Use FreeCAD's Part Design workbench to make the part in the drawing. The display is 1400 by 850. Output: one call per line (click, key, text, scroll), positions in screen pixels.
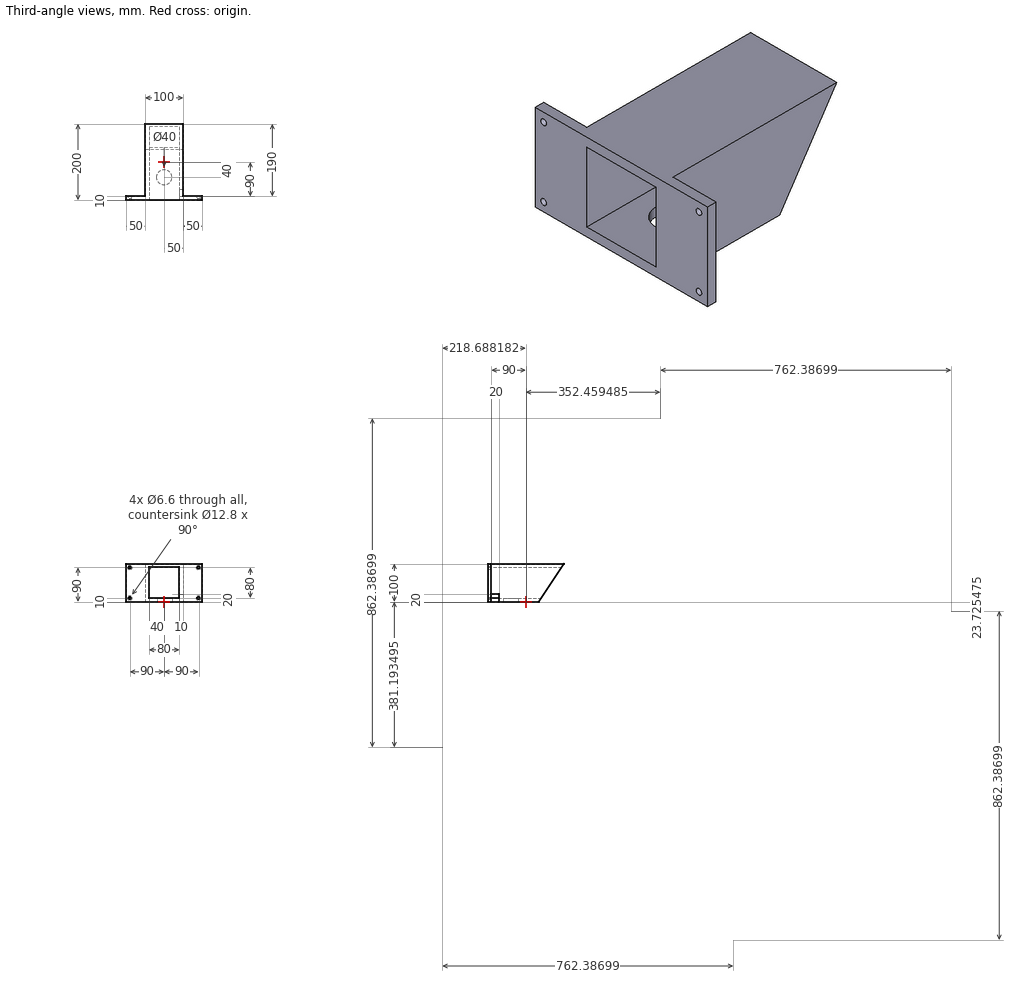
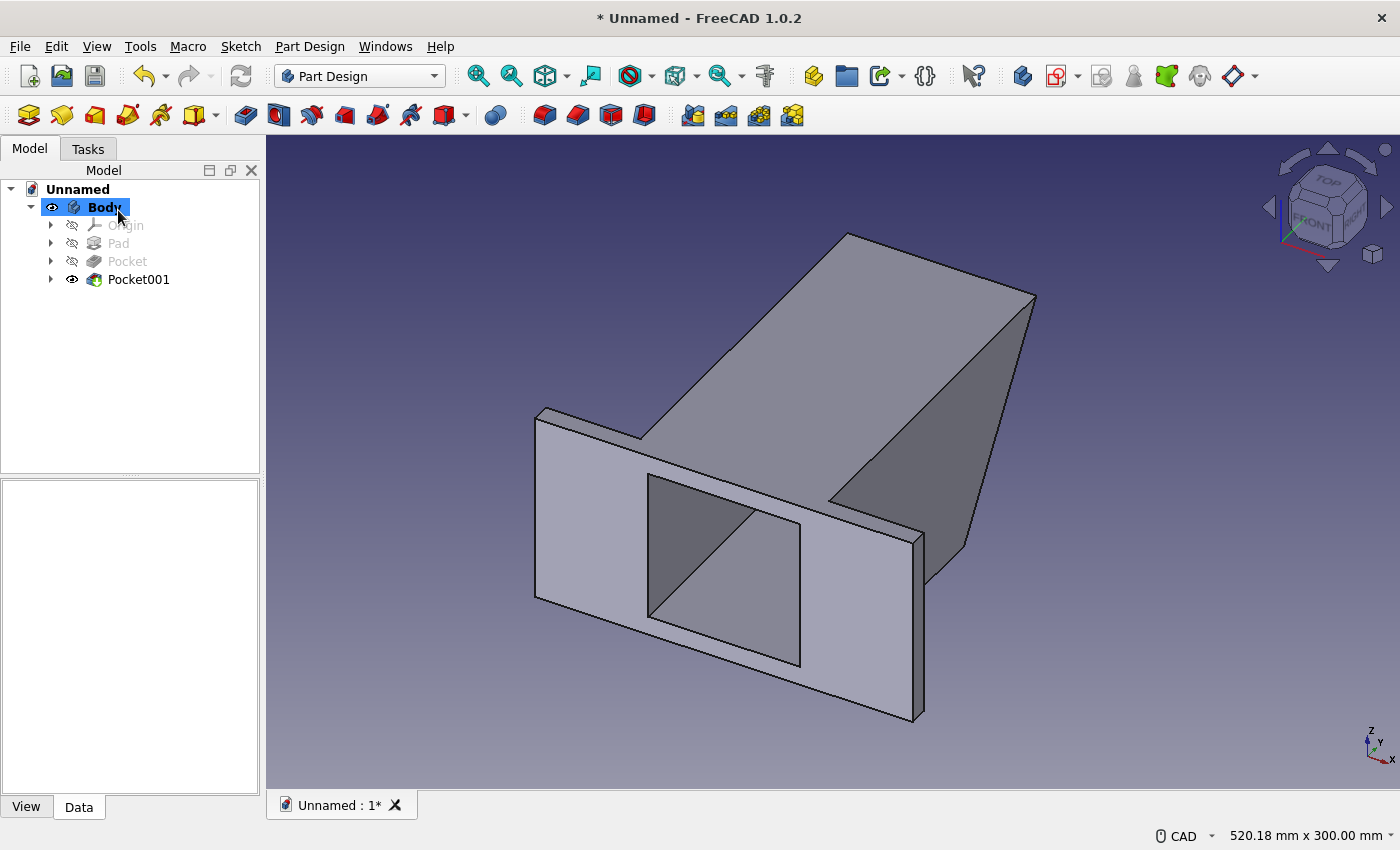
key(5)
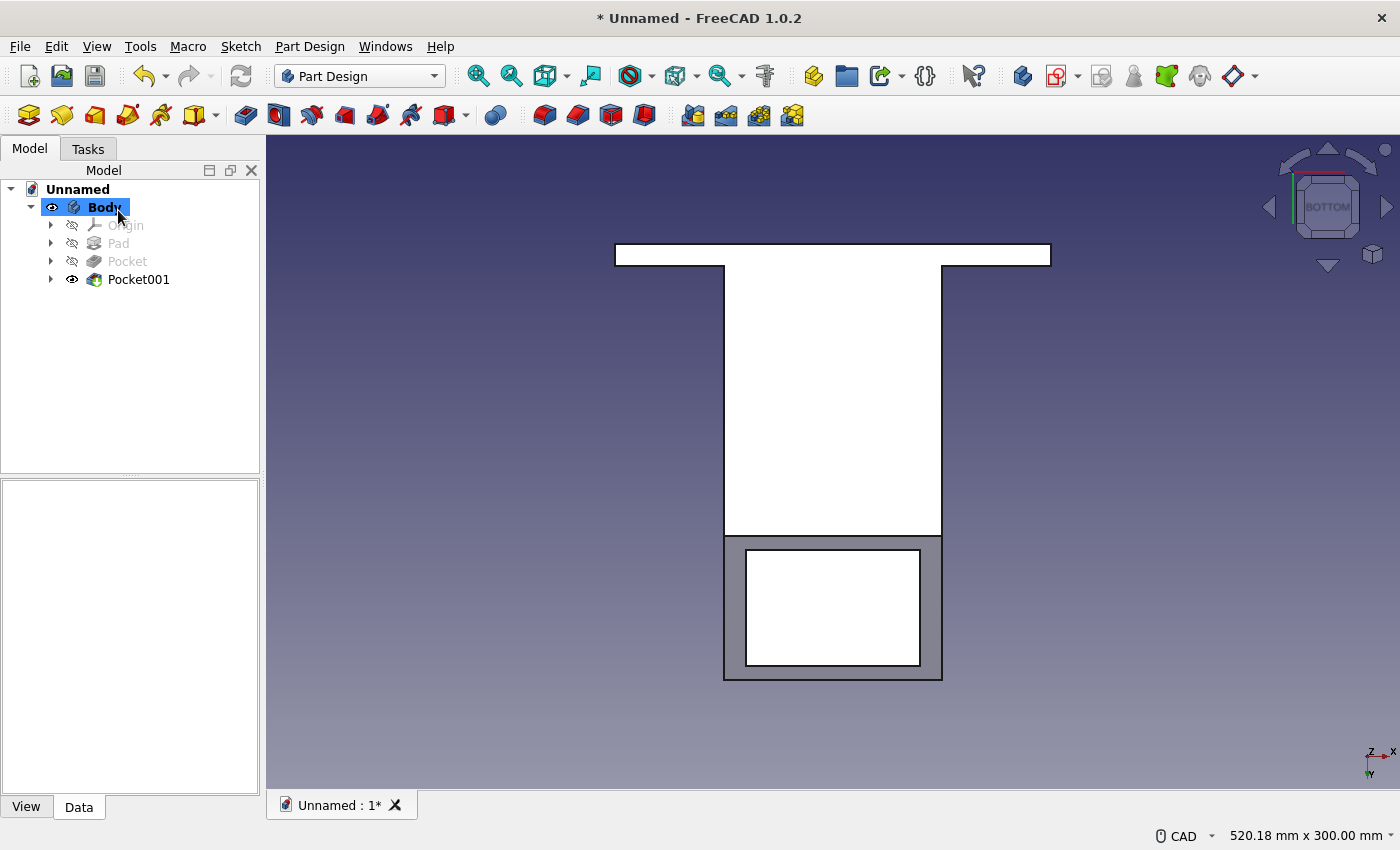
click(833, 389)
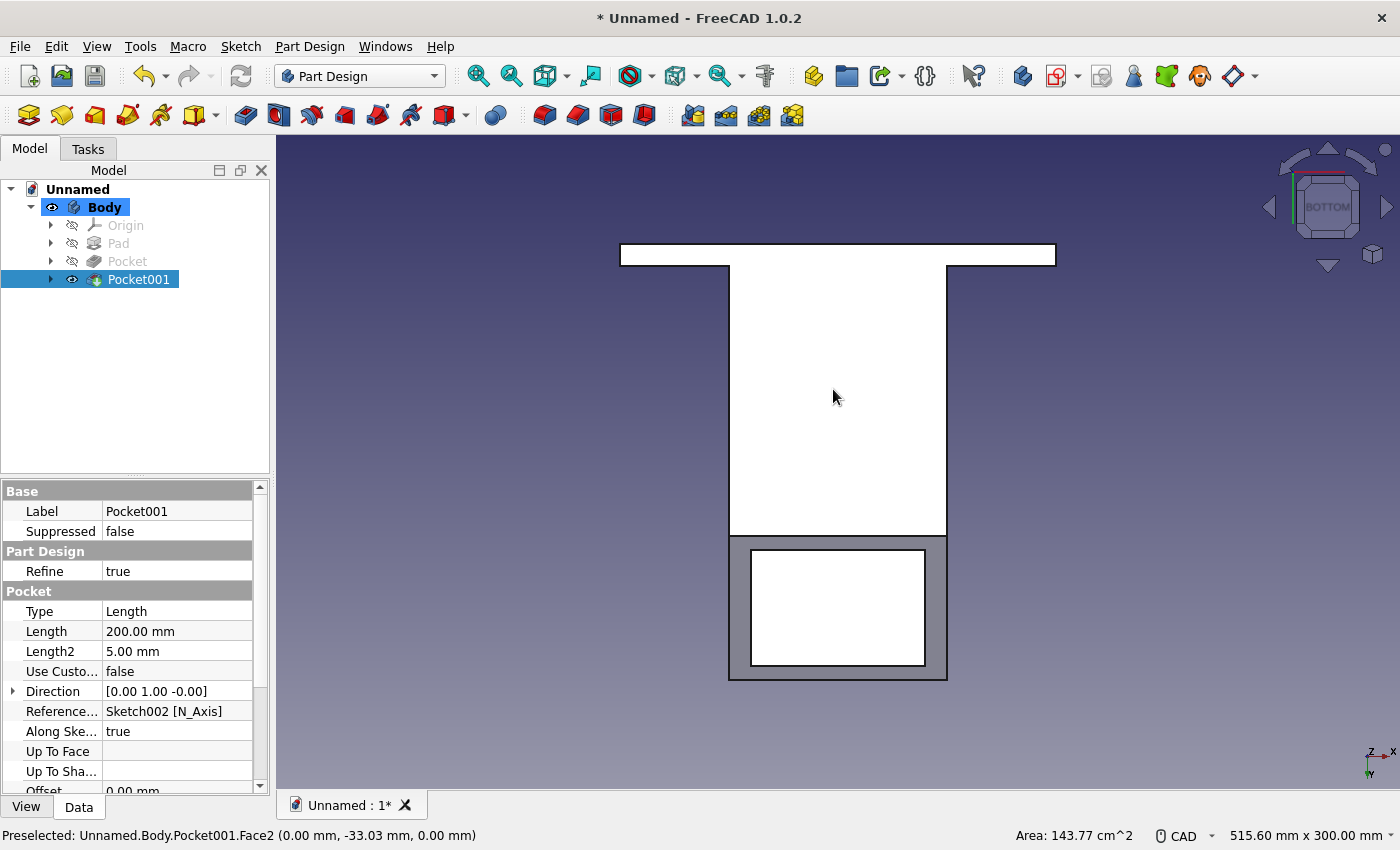
click(1056, 76)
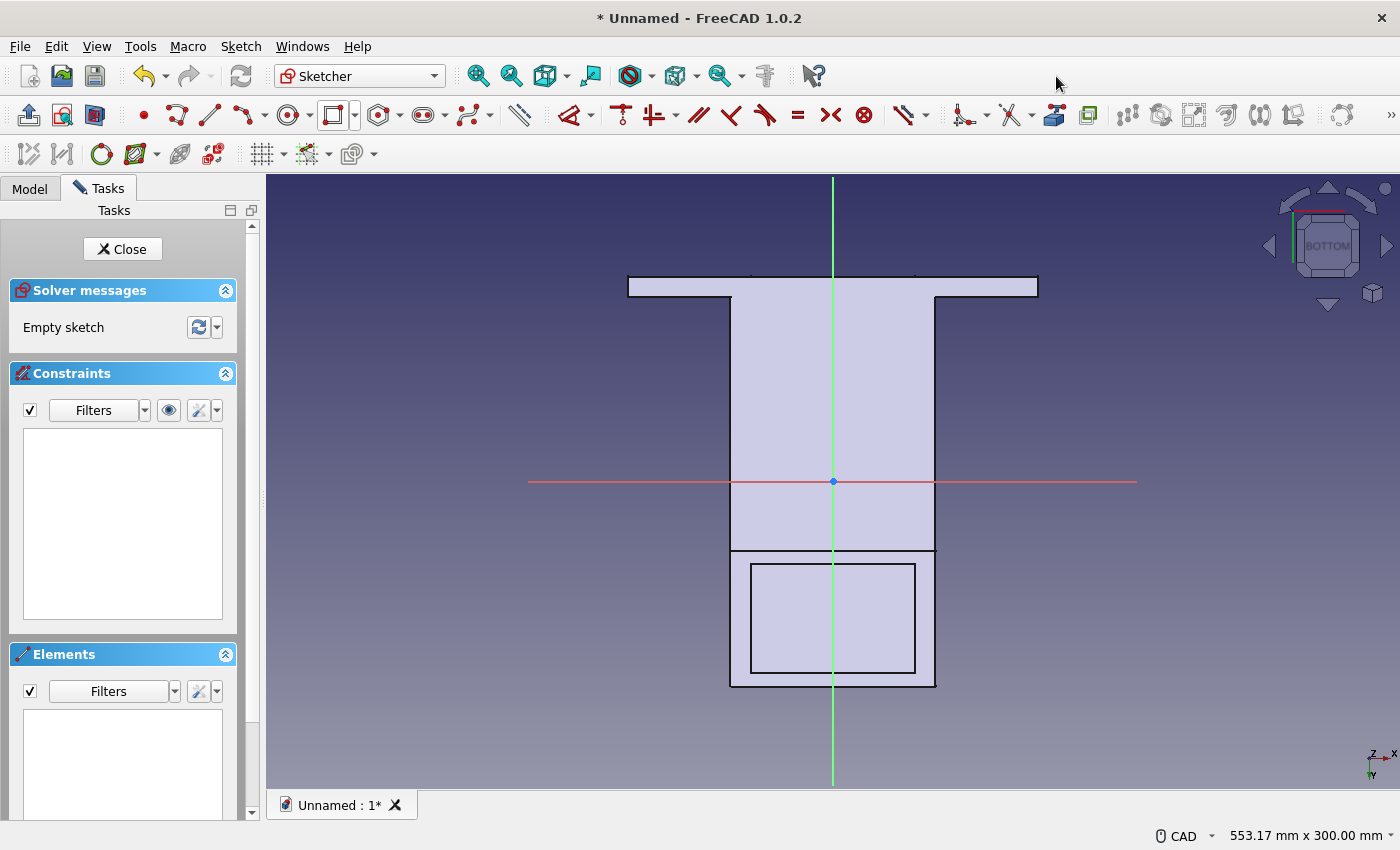
scroll(863, 393, up, 6)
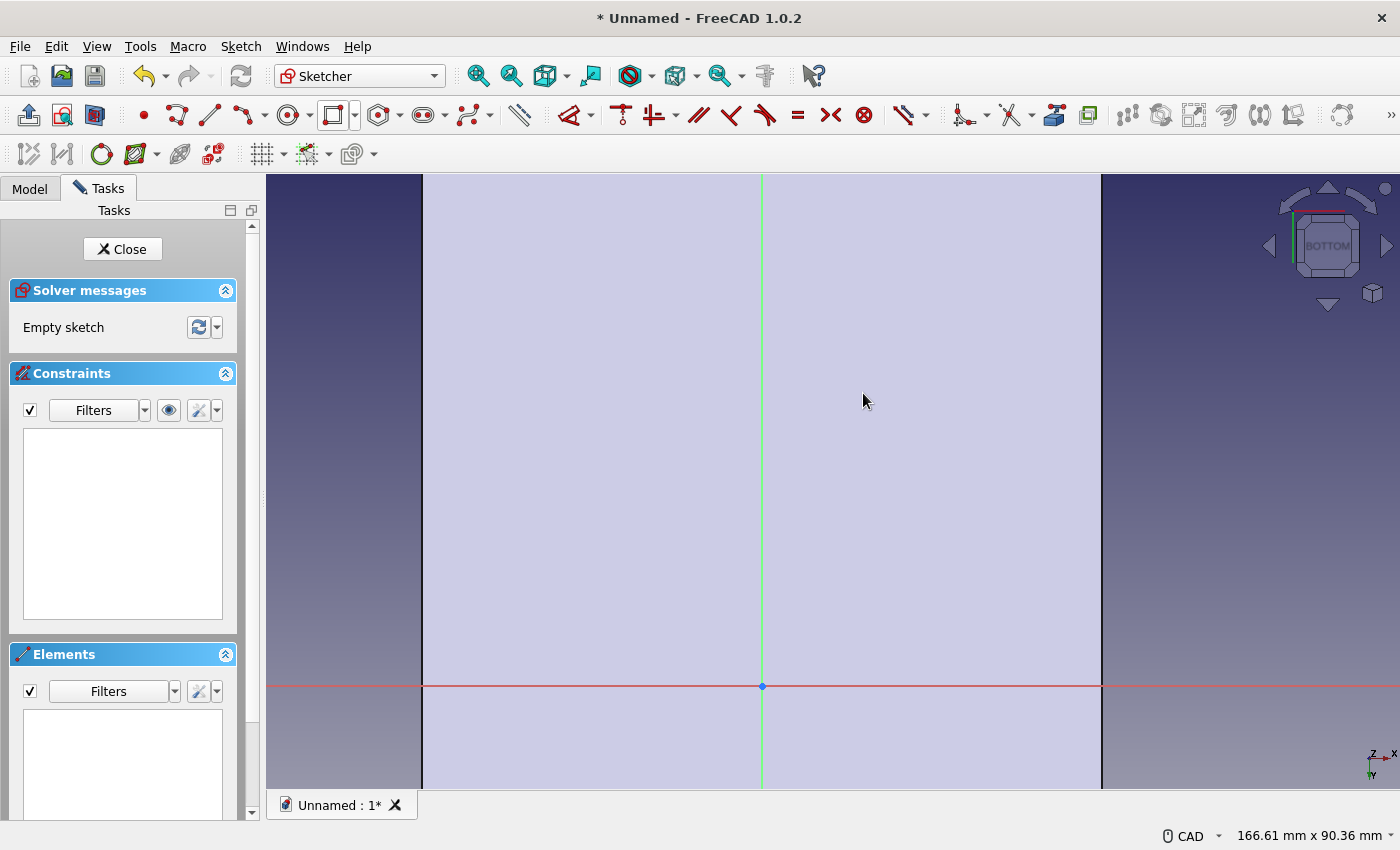
key(g)
key(c)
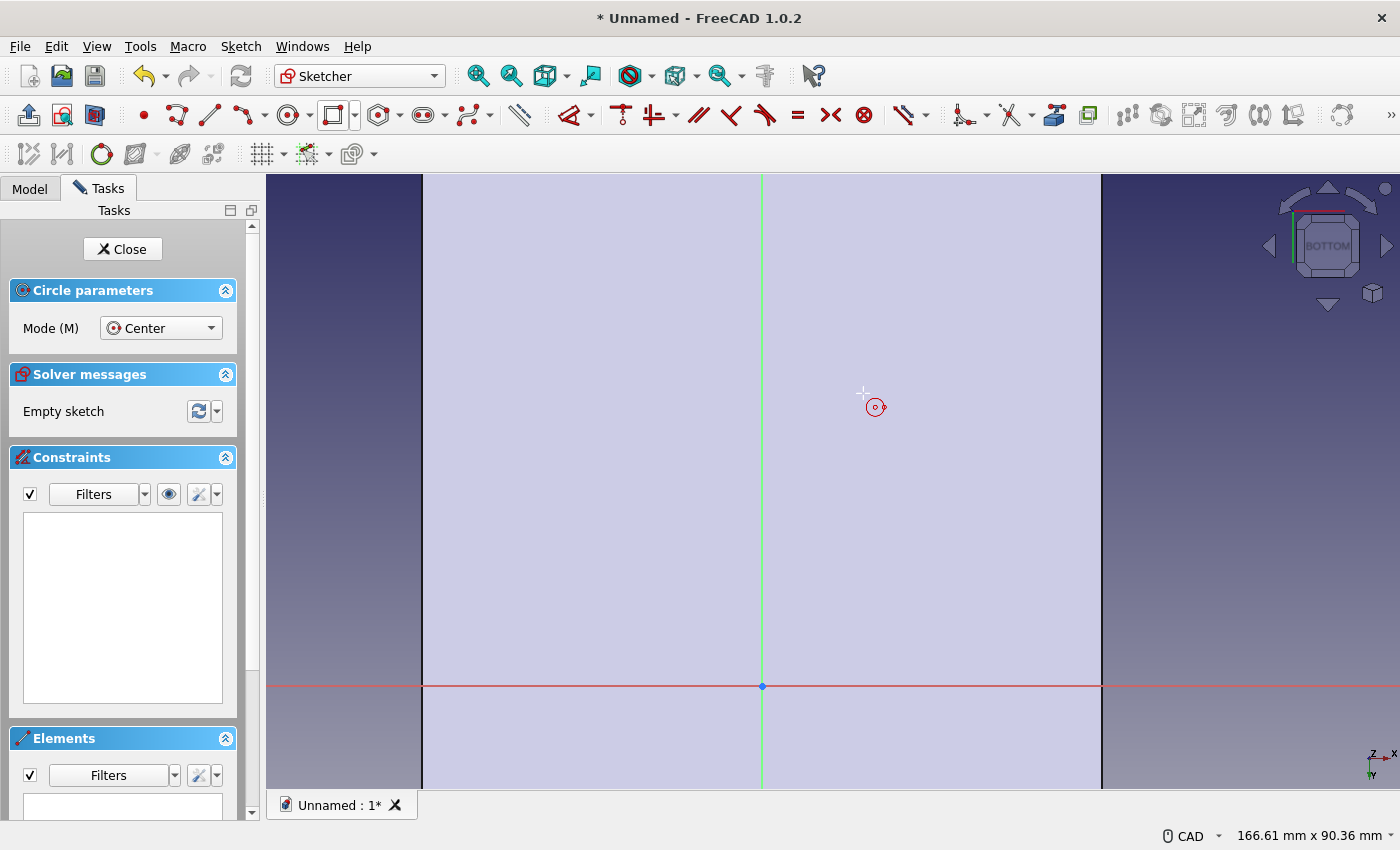
click(762, 414)
move(858, 317)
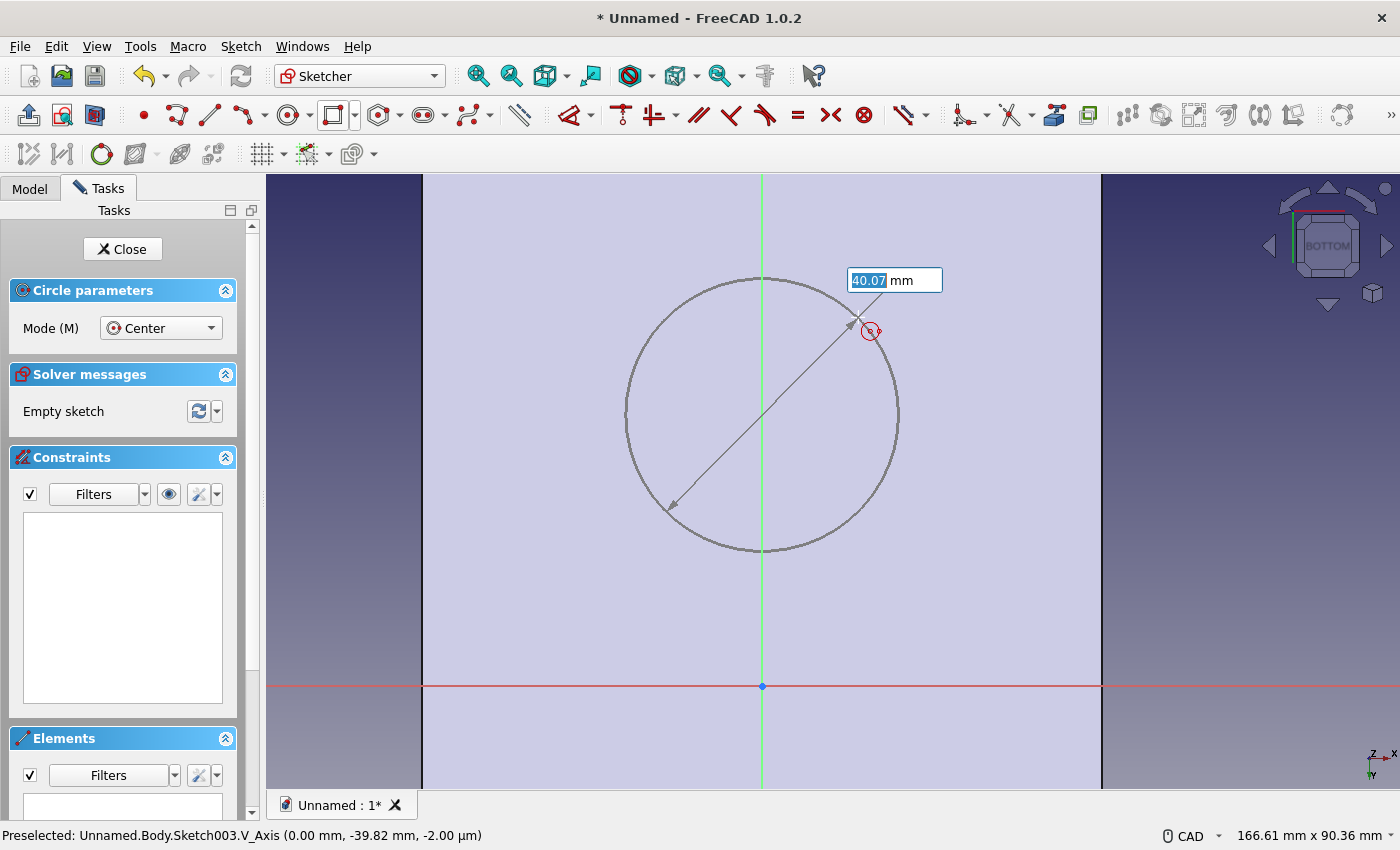
text(40)
key(Return)
key(Escape)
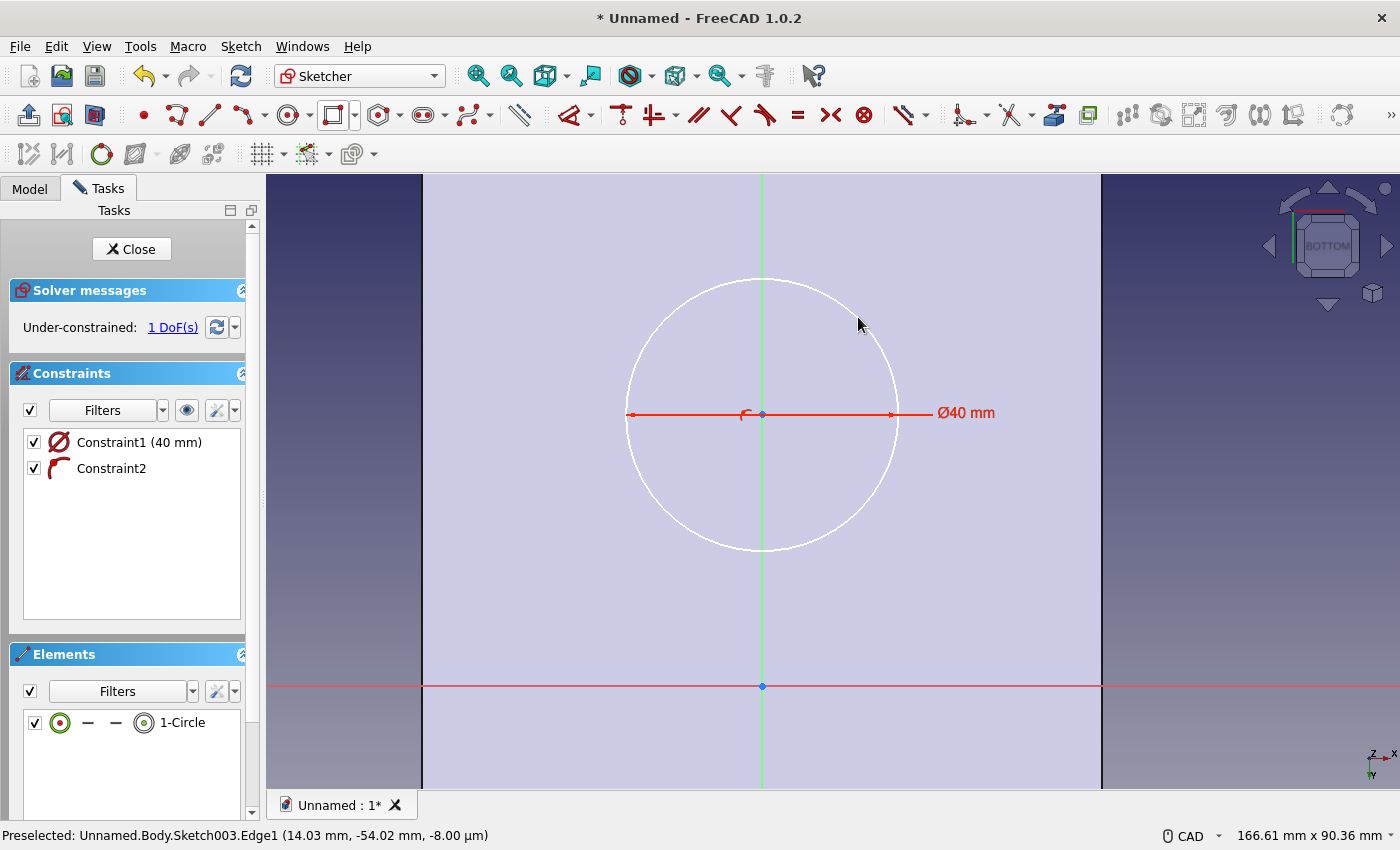
key(d)